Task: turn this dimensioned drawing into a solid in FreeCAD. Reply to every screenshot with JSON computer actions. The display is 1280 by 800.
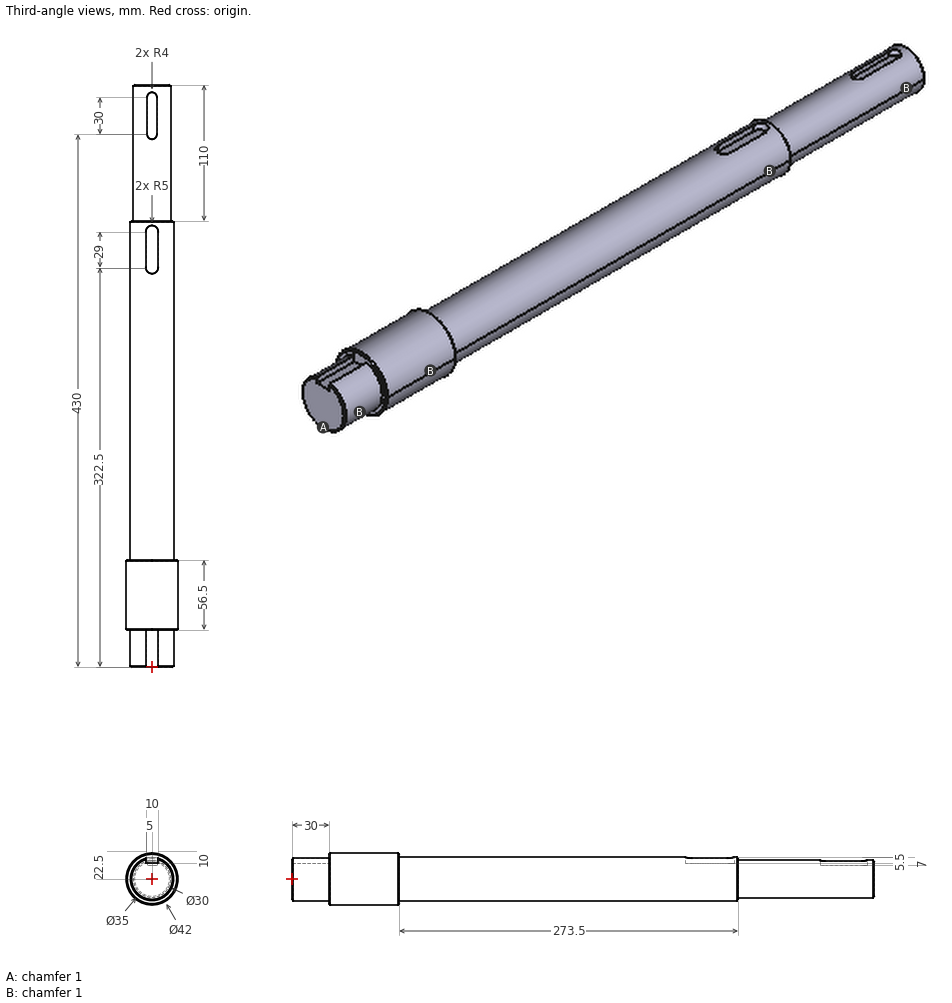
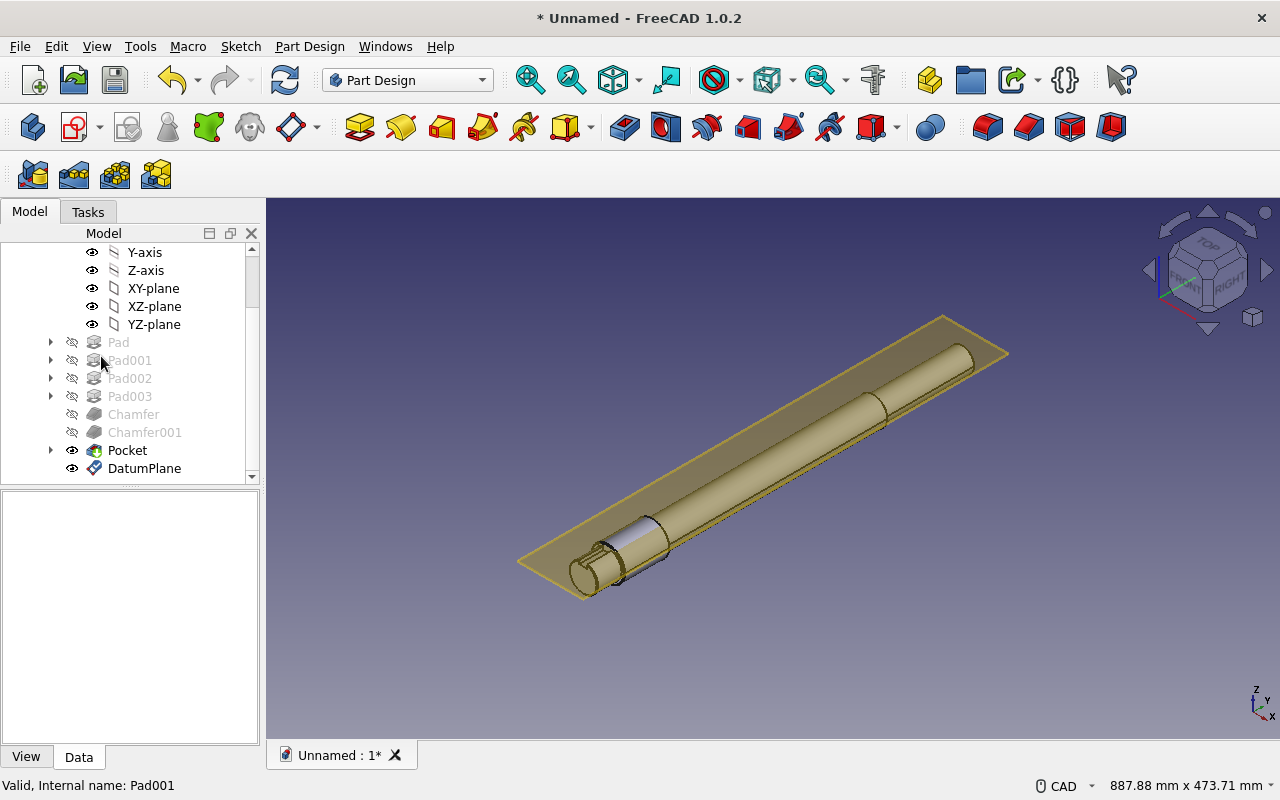
{"action": "left_click", "coordinate": [117, 468]}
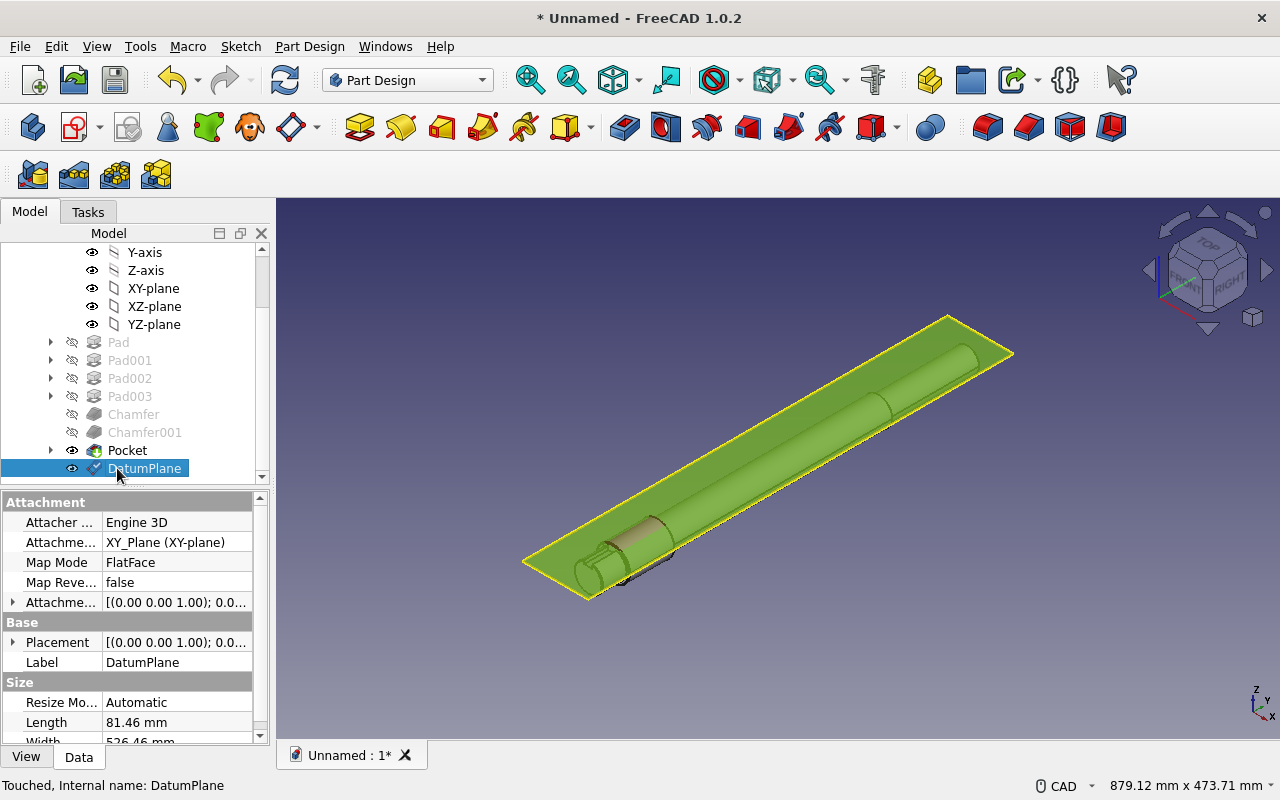
{"action": "left_click", "coordinate": [74, 128]}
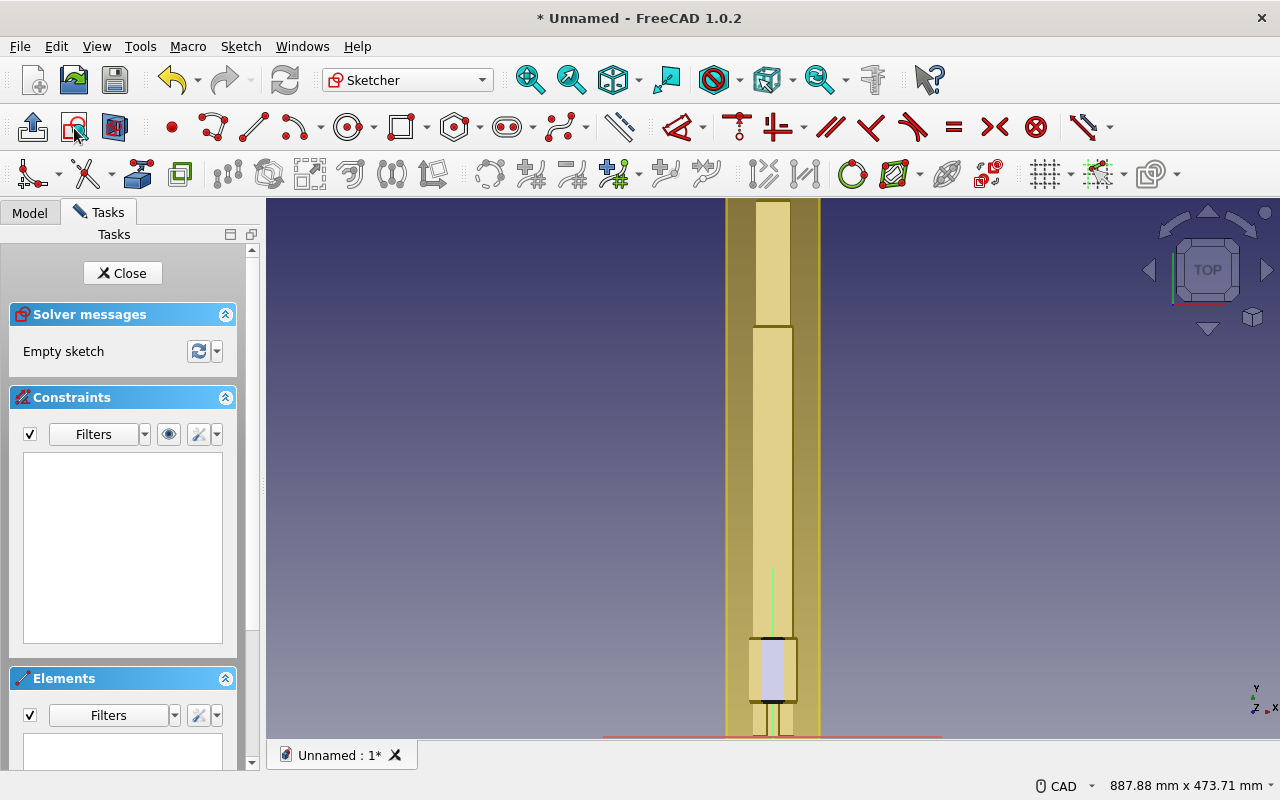
{"action": "key", "text": "q s"}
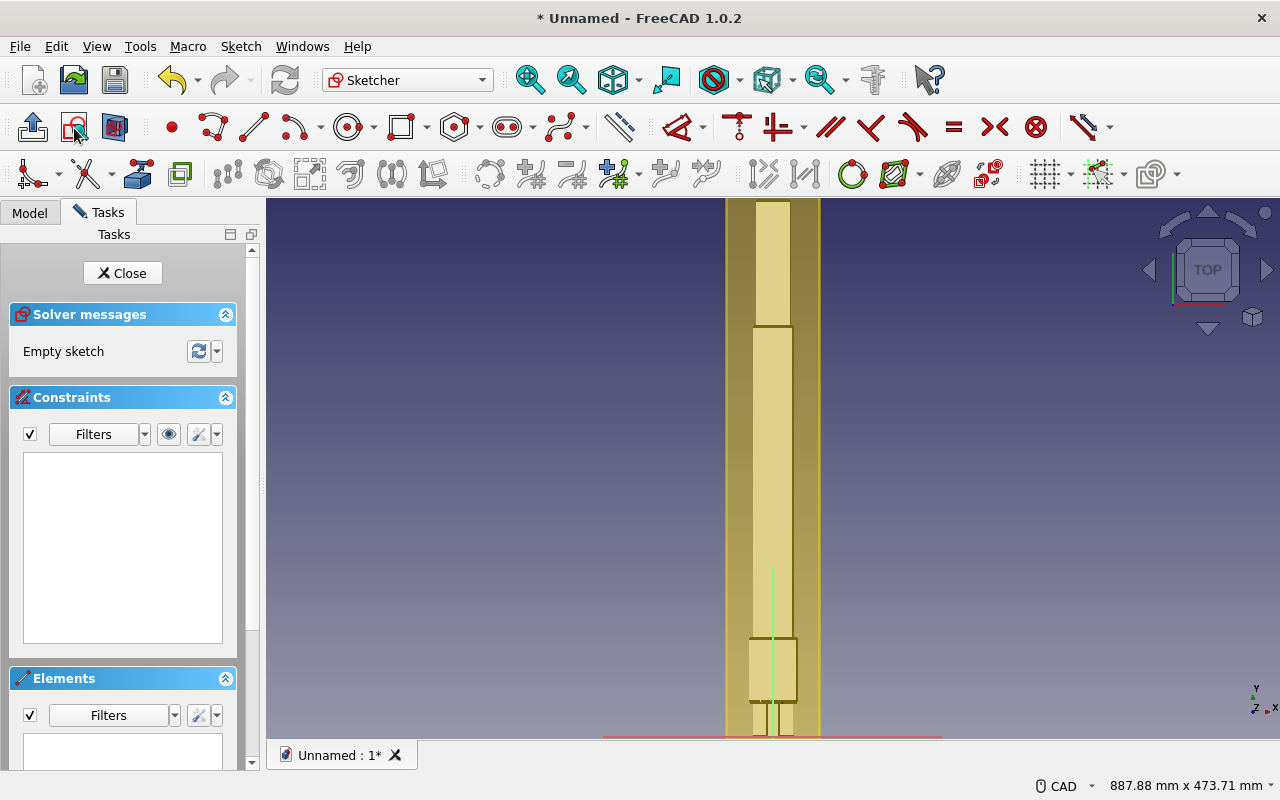
{"action": "scroll", "coordinate": [784, 334], "scroll_direction": "up", "scroll_amount": 10}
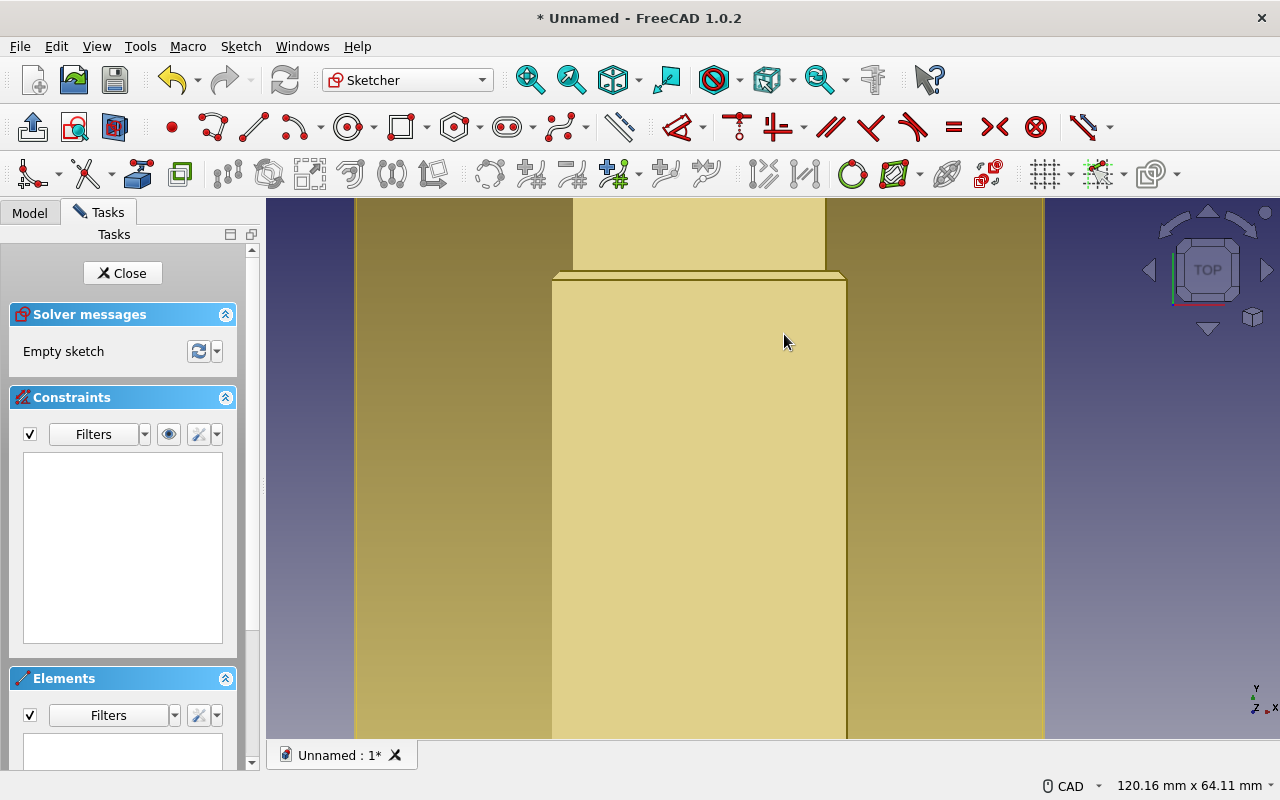
{"action": "left_click", "coordinate": [506, 128]}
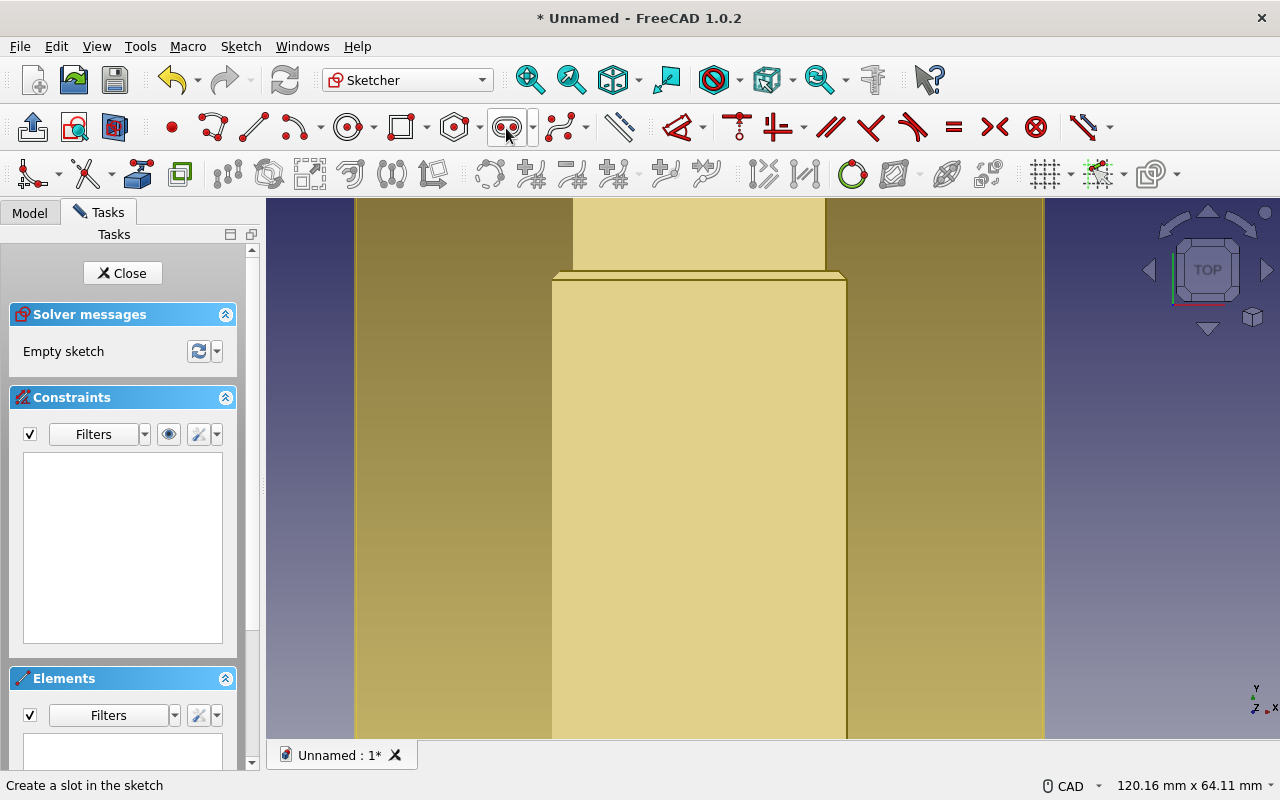
{"action": "left_click", "coordinate": [699, 588]}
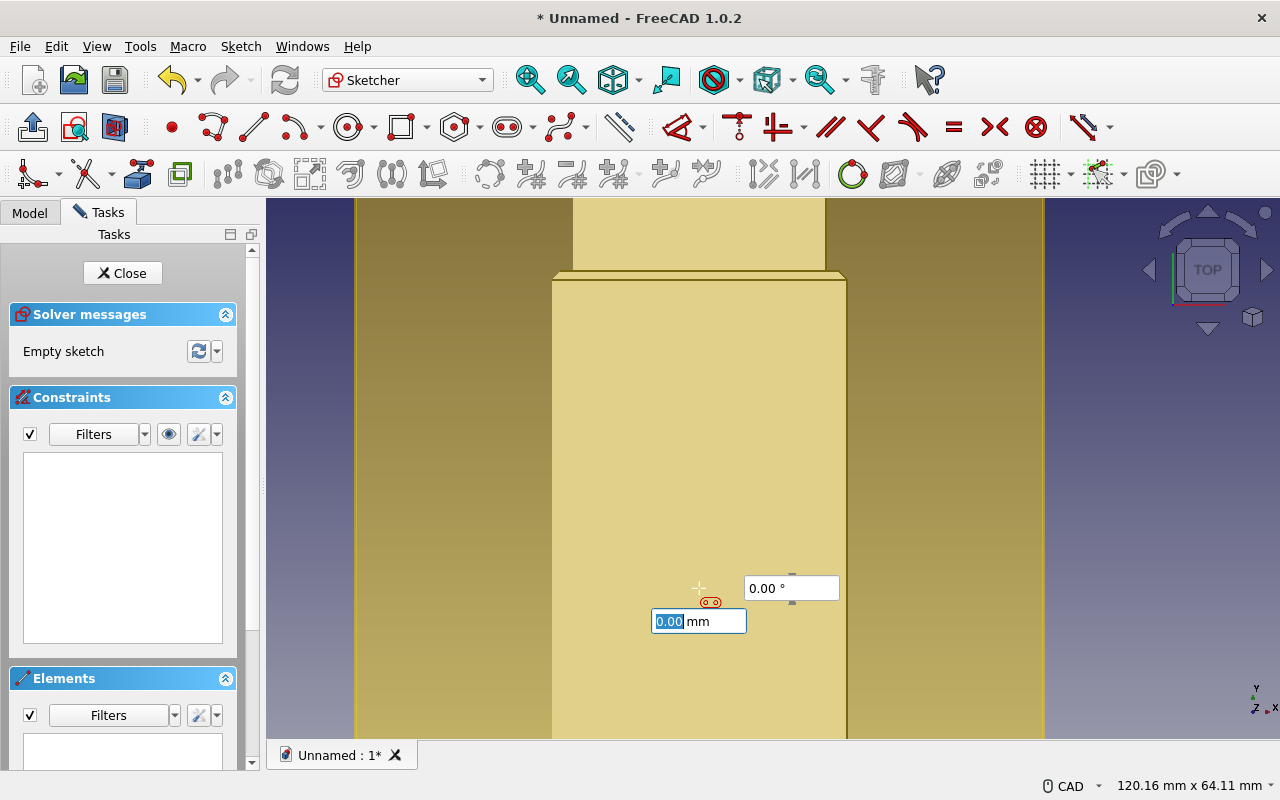
{"action": "left_click", "coordinate": [708, 343]}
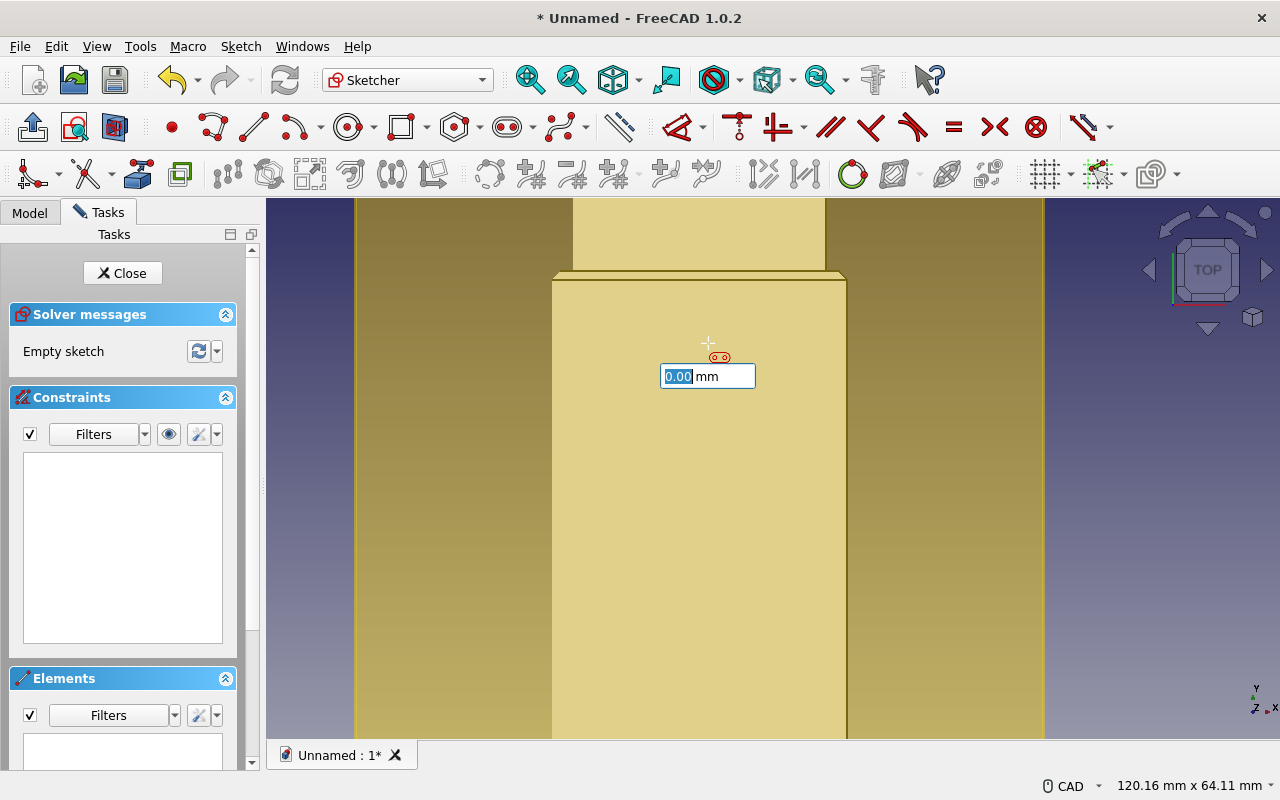
{"action": "left_click", "coordinate": [742, 465]}
{"action": "key", "text": "Escape"}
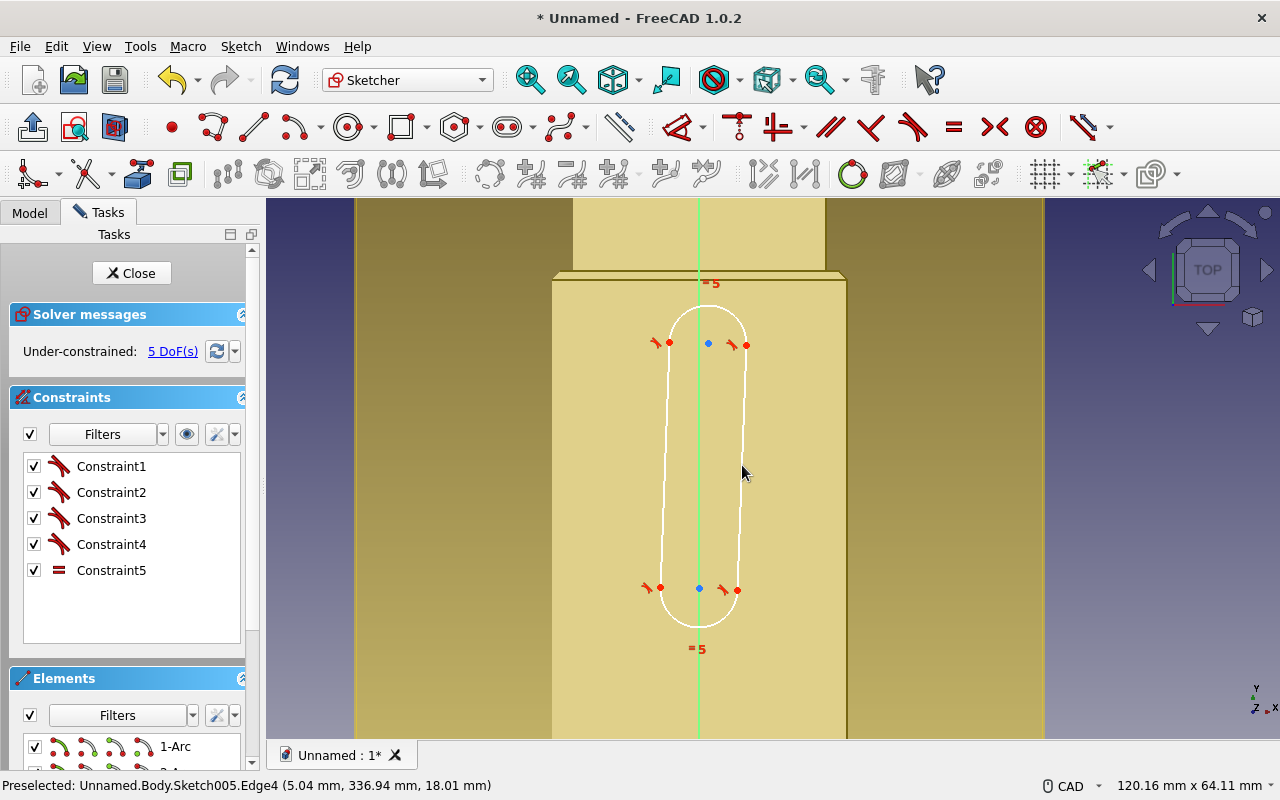
{"action": "left_click", "coordinate": [663, 514]}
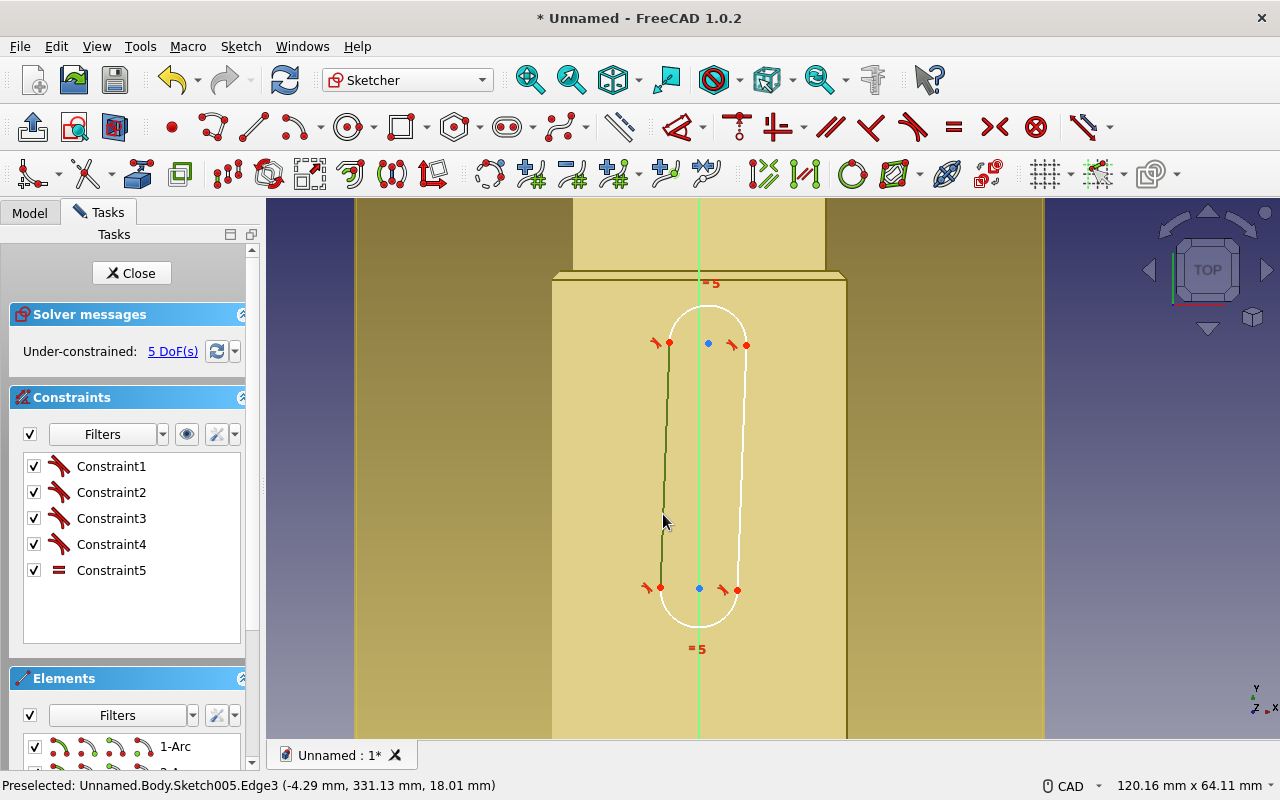
{"action": "key", "text": "v"}